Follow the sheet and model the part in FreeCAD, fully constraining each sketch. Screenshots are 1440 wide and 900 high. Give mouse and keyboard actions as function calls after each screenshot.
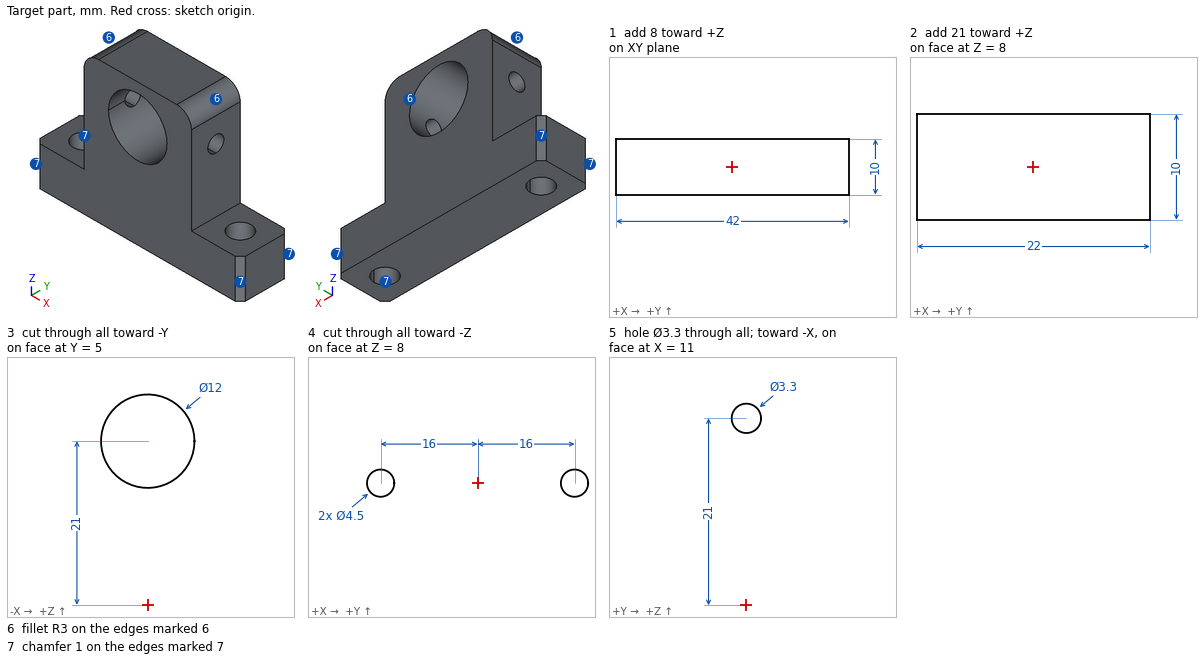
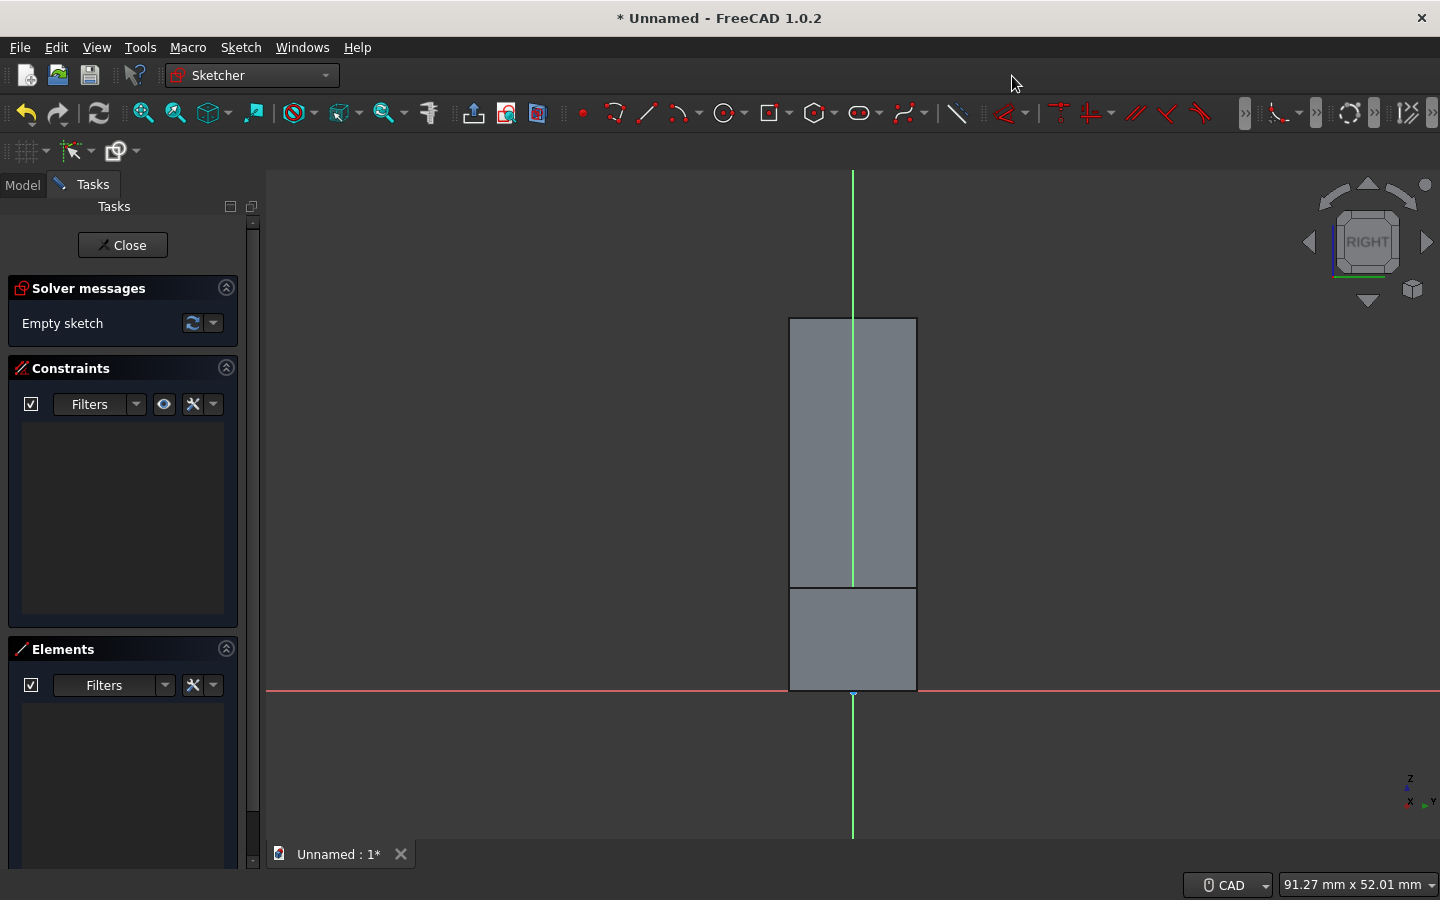
click(538, 114)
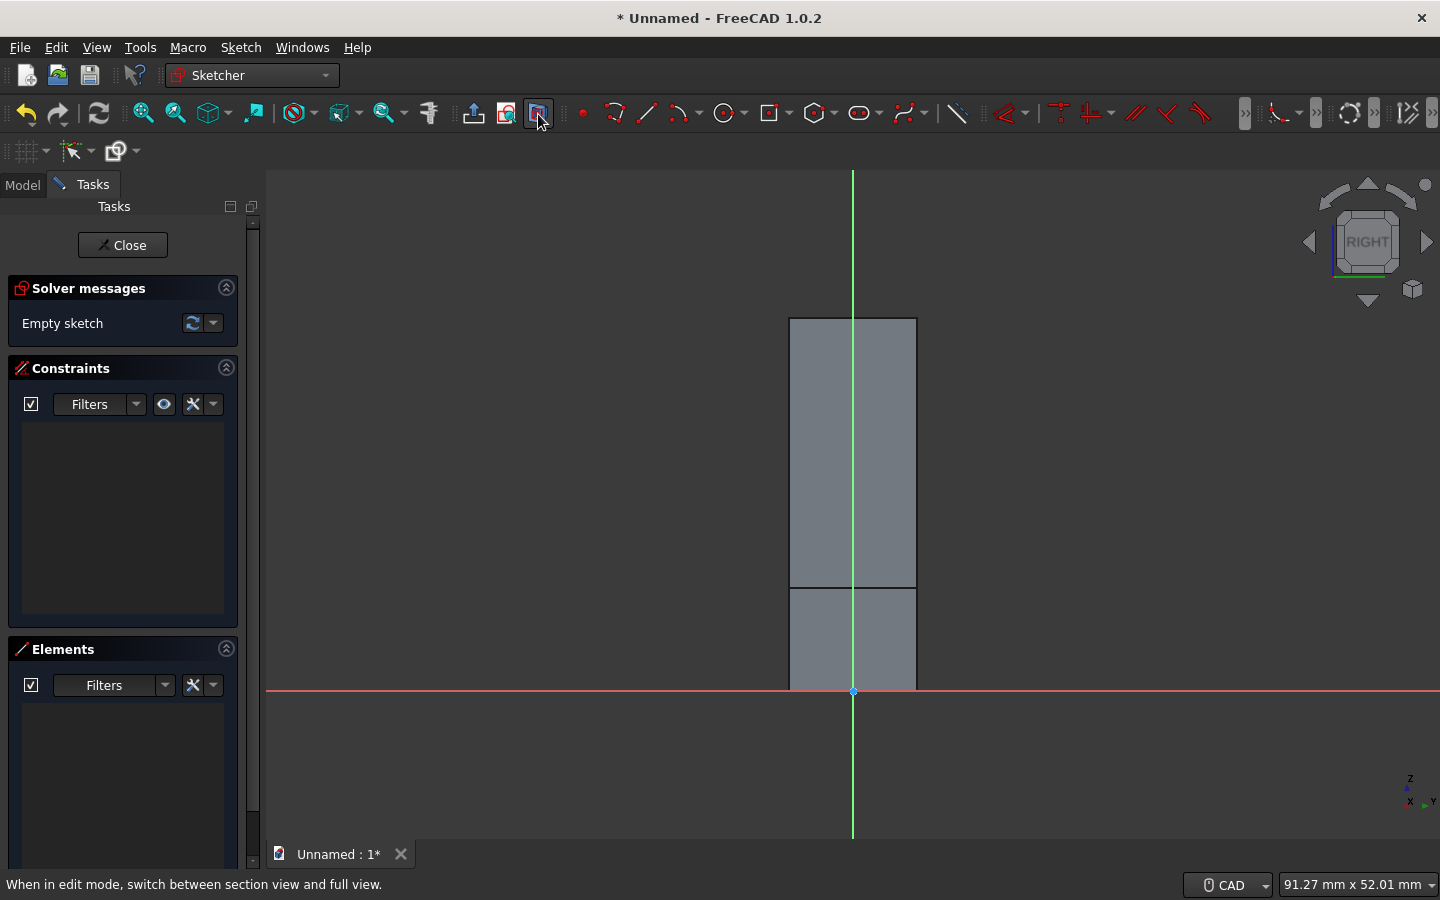
scroll(860, 413, up, 12)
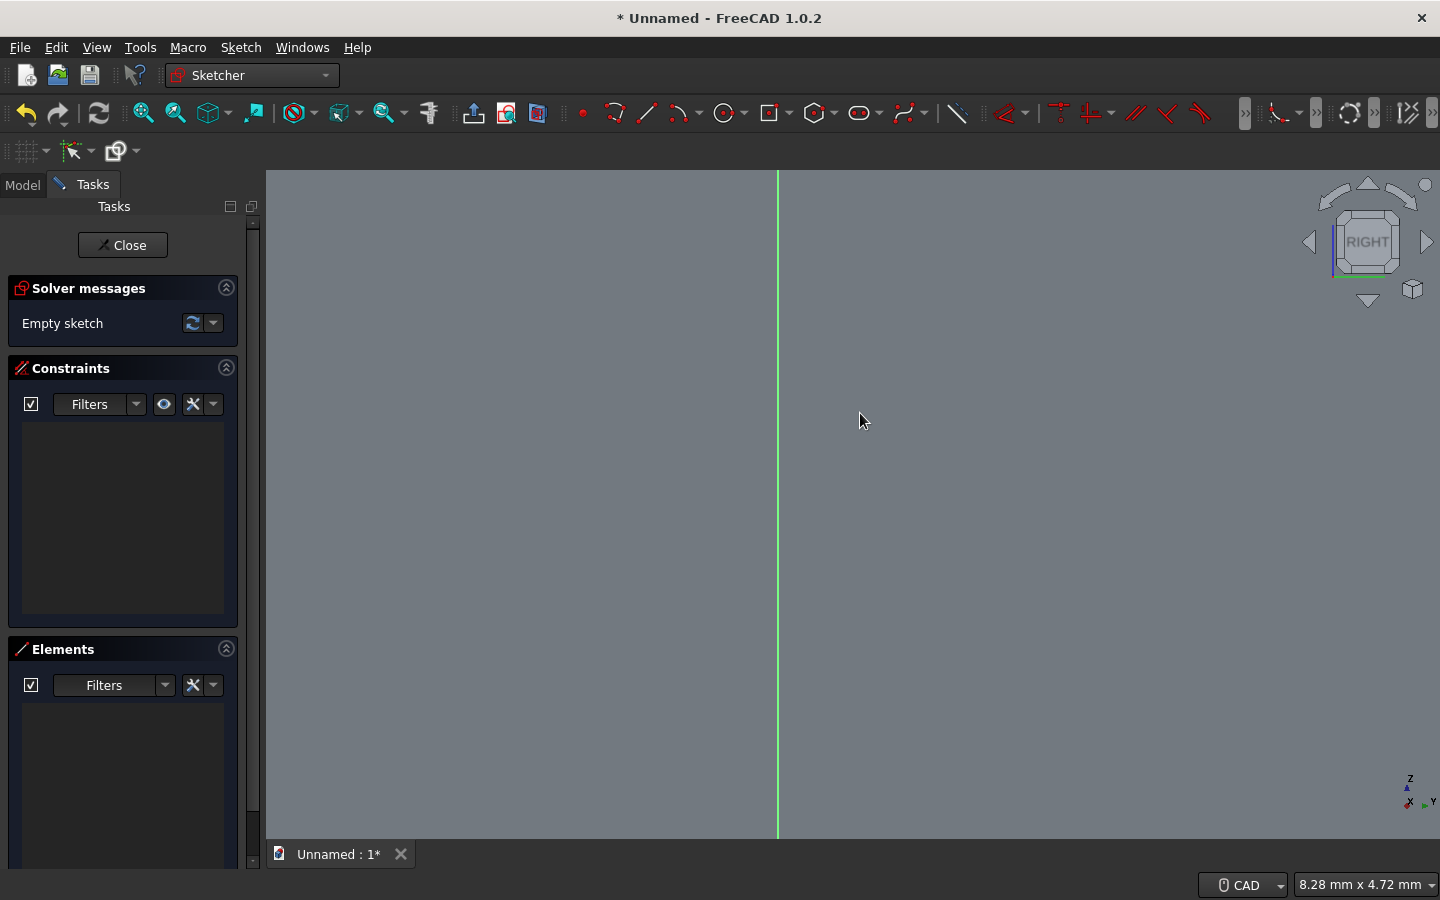
click(724, 114)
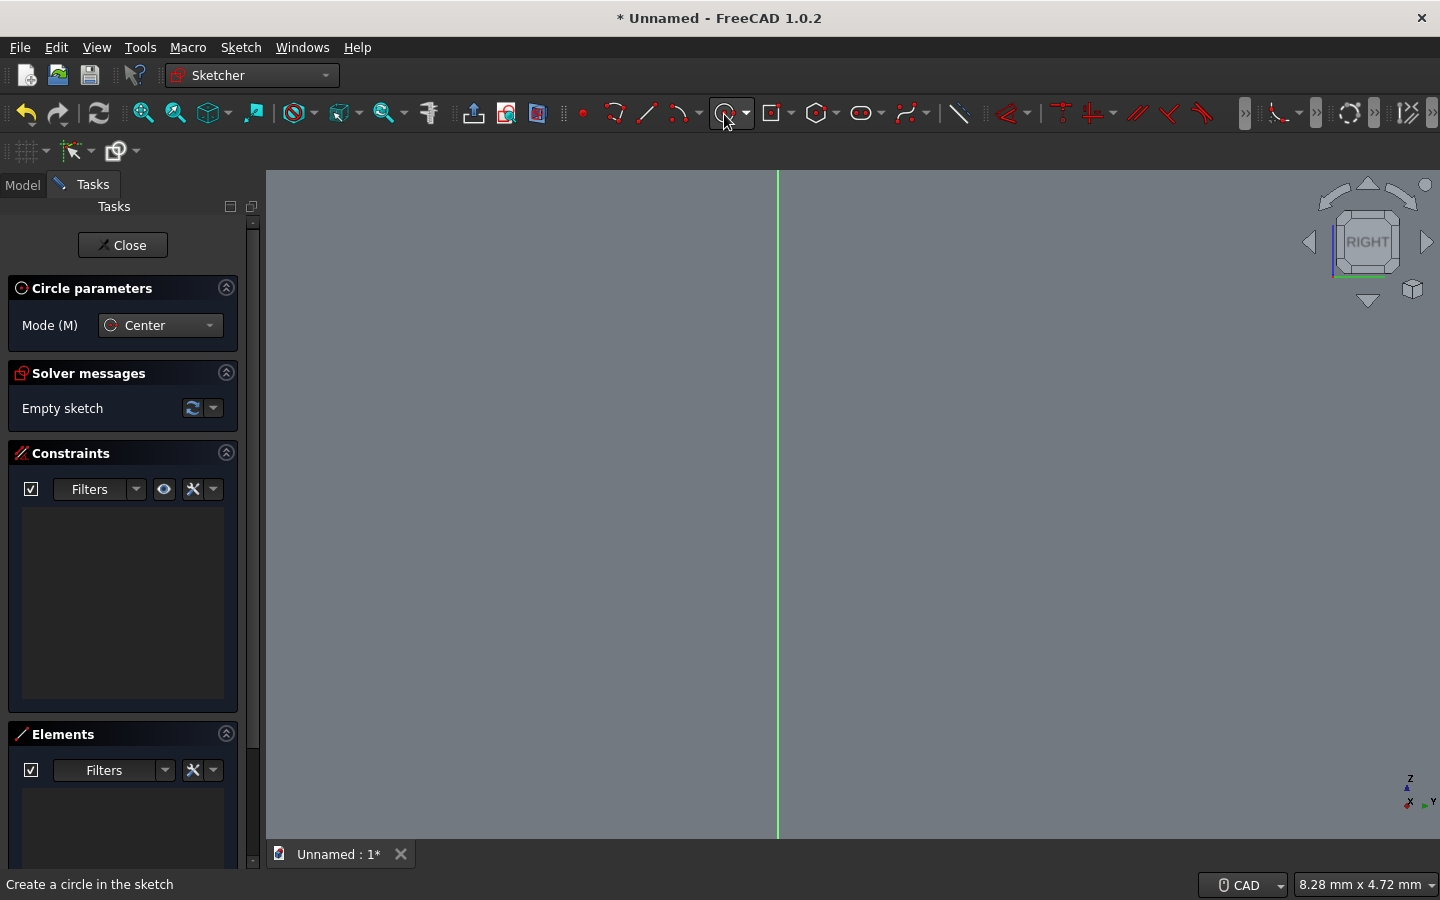
click(778, 496)
click(943, 331)
key(Escape)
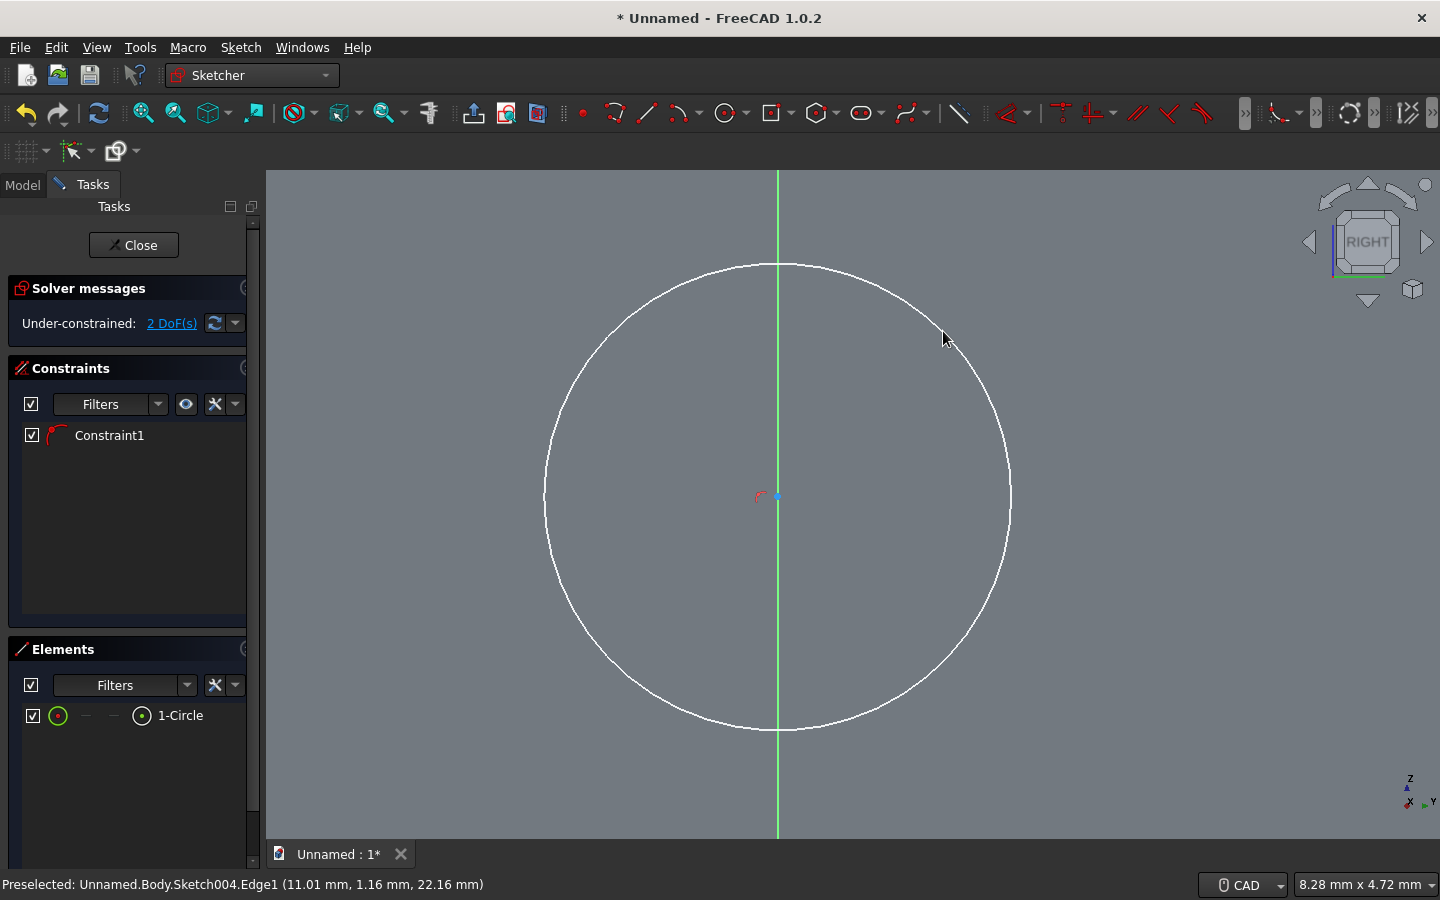
click(1006, 114)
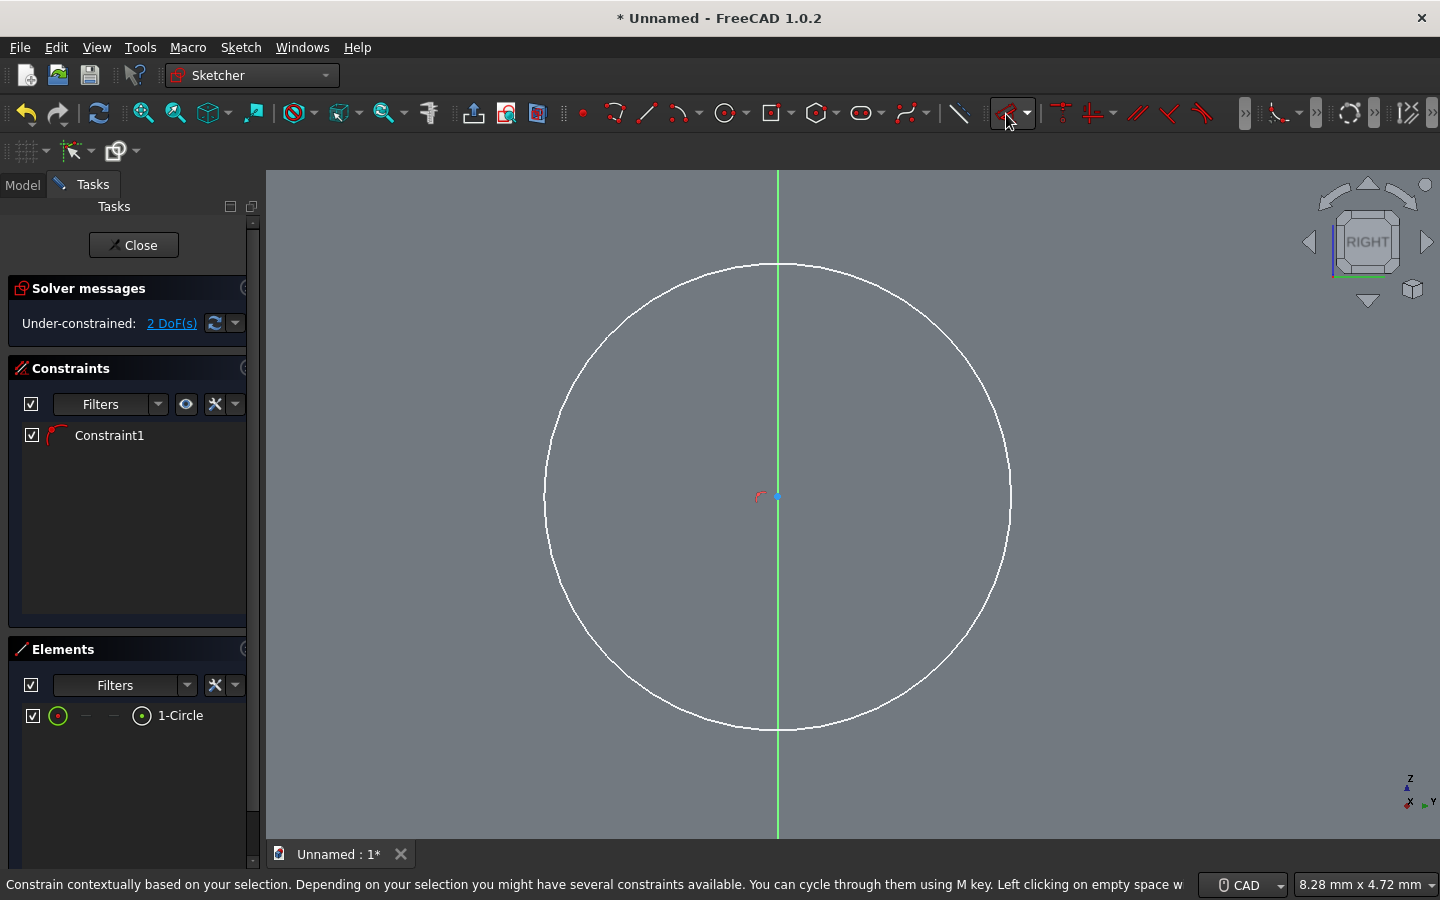
click(942, 331)
click(965, 308)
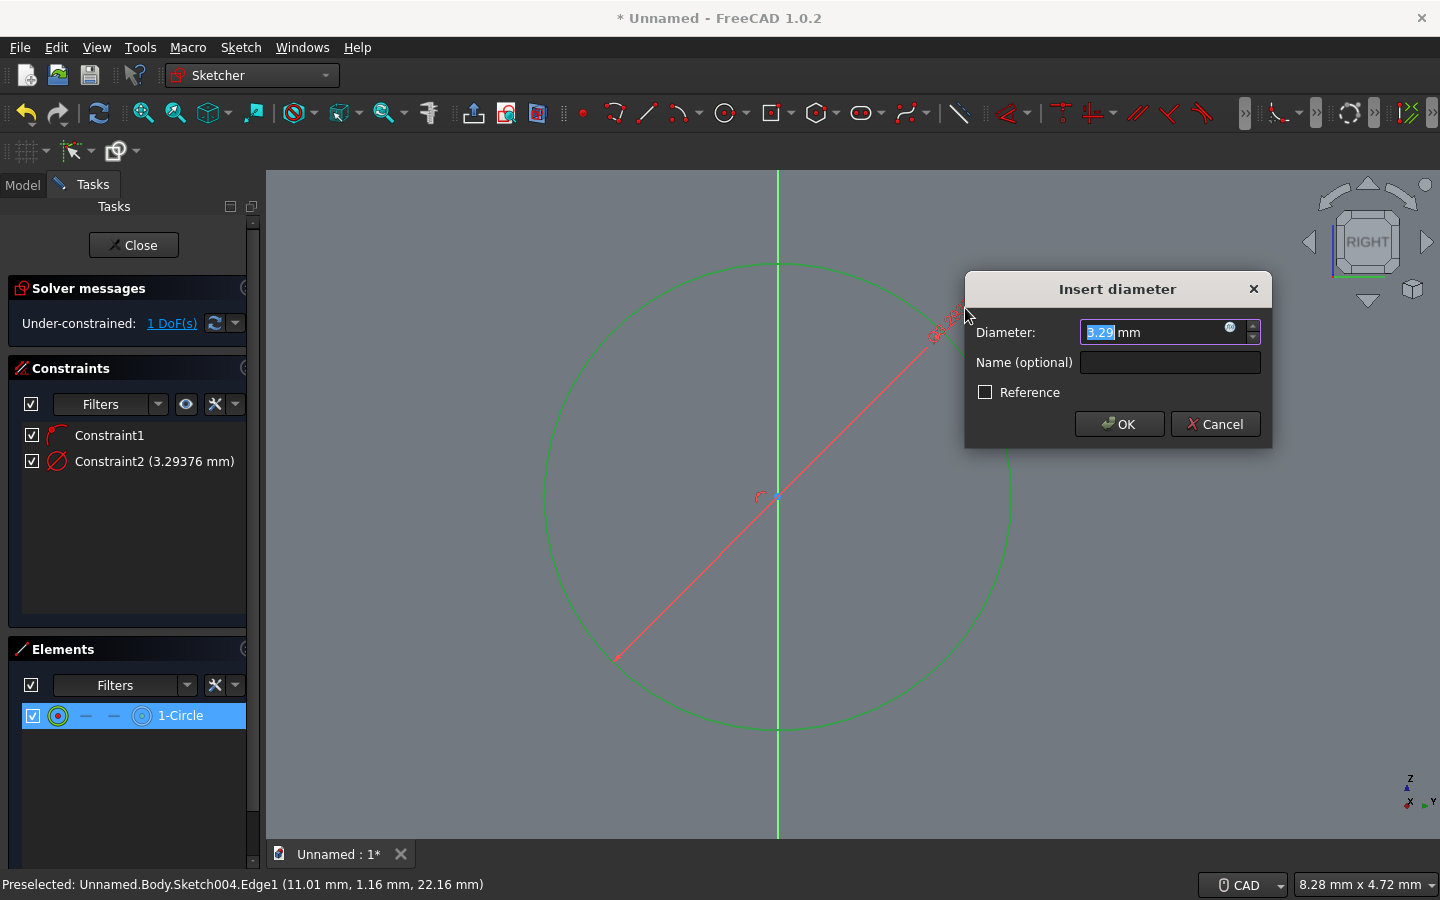
text(3.3)
key(Return)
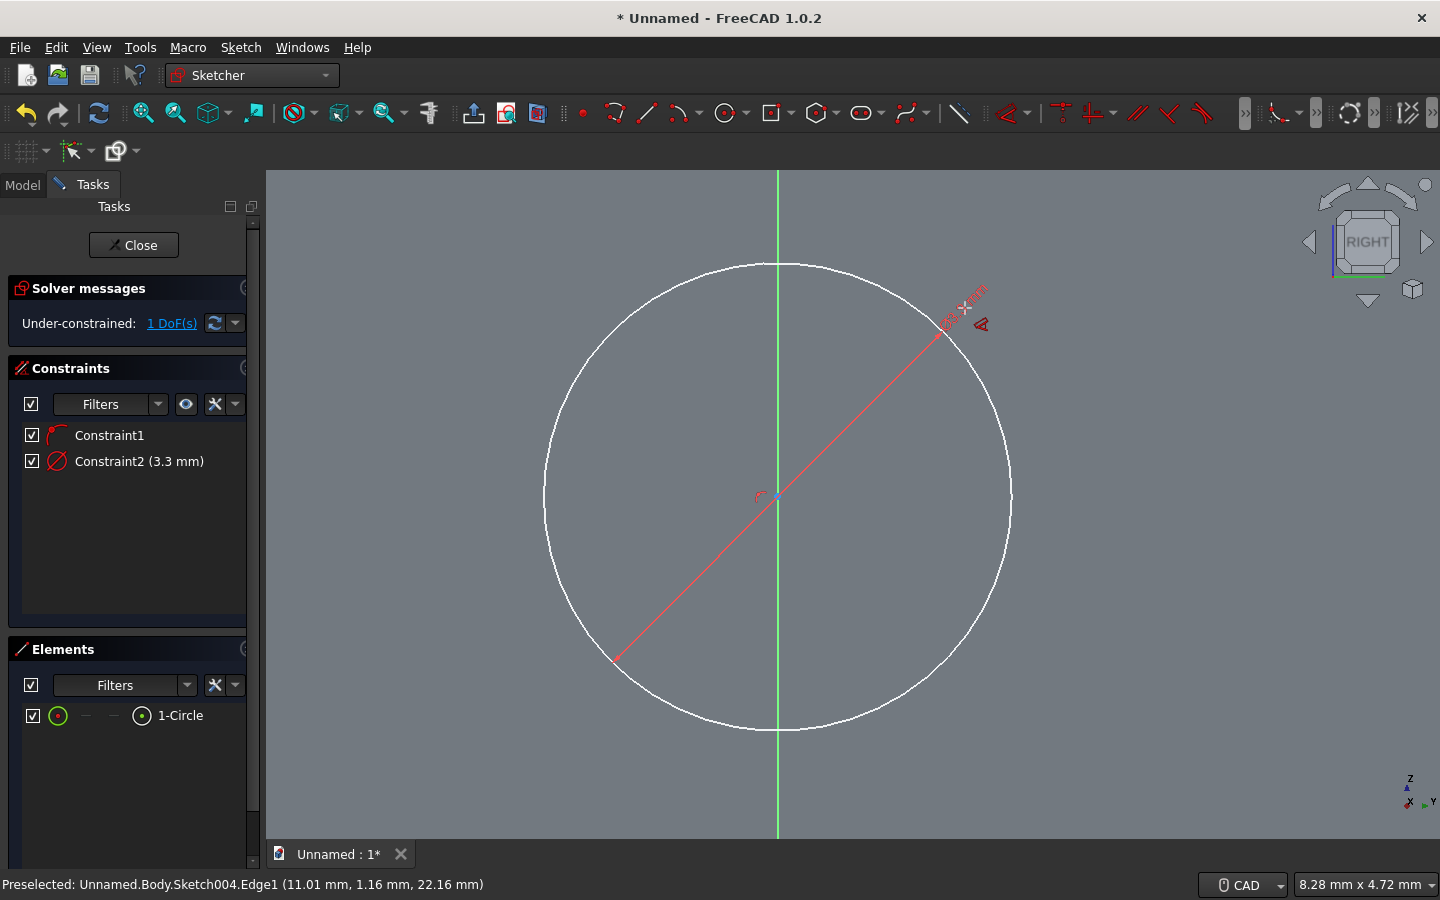
click(778, 497)
click(812, 654)